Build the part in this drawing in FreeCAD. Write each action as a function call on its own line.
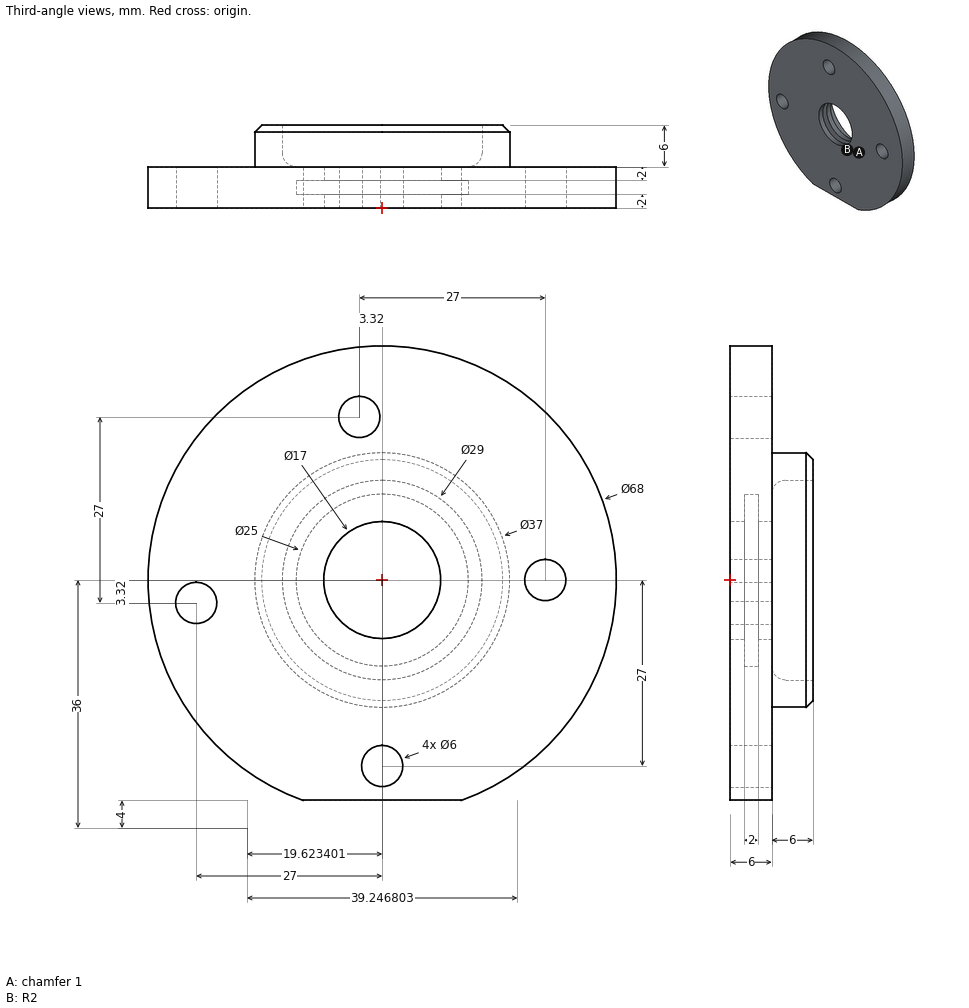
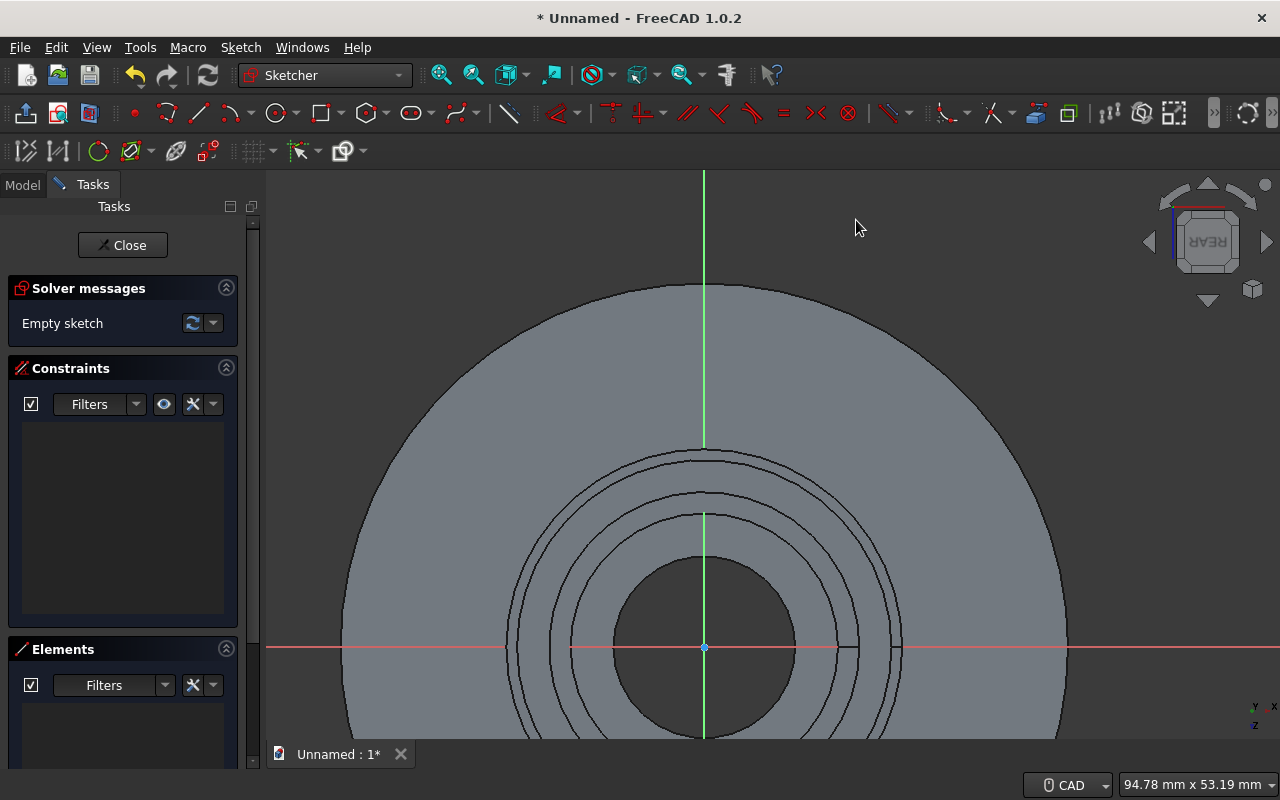
click(322, 114)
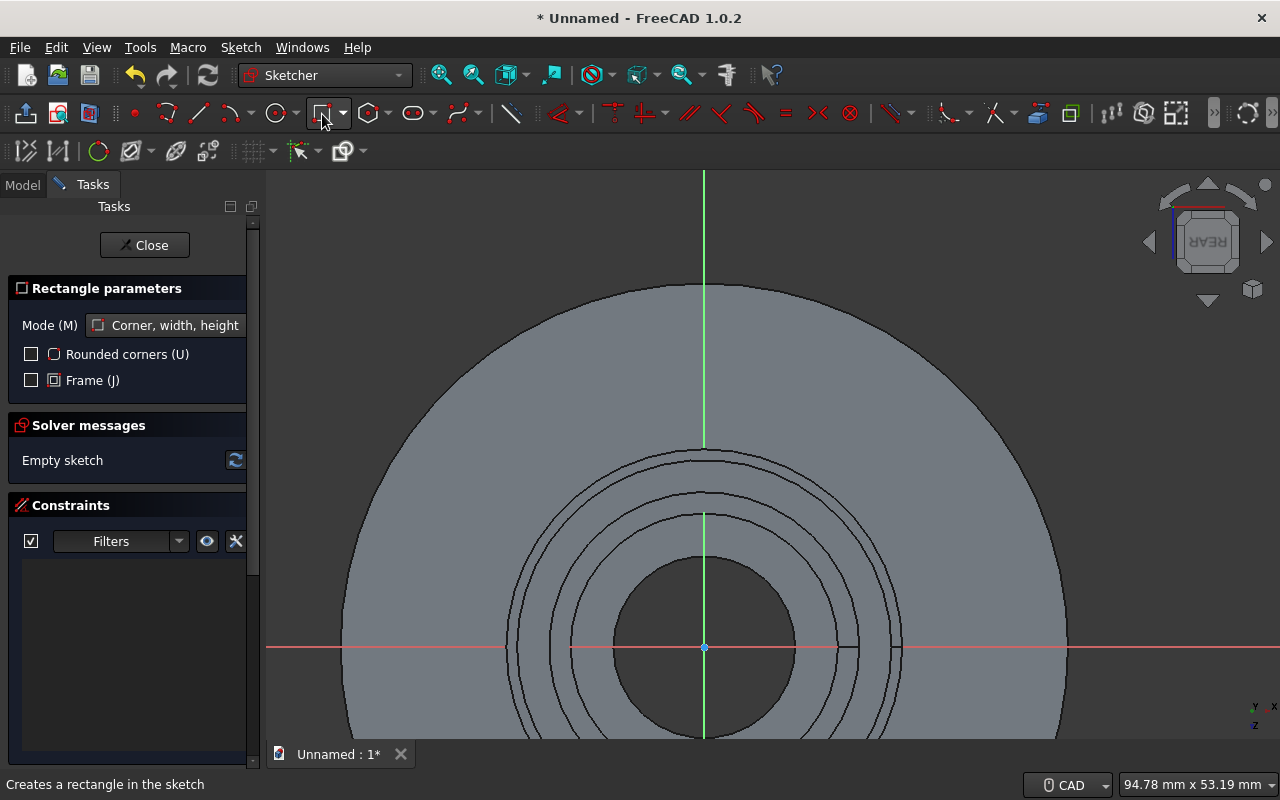
click(494, 262)
click(914, 305)
key(Escape)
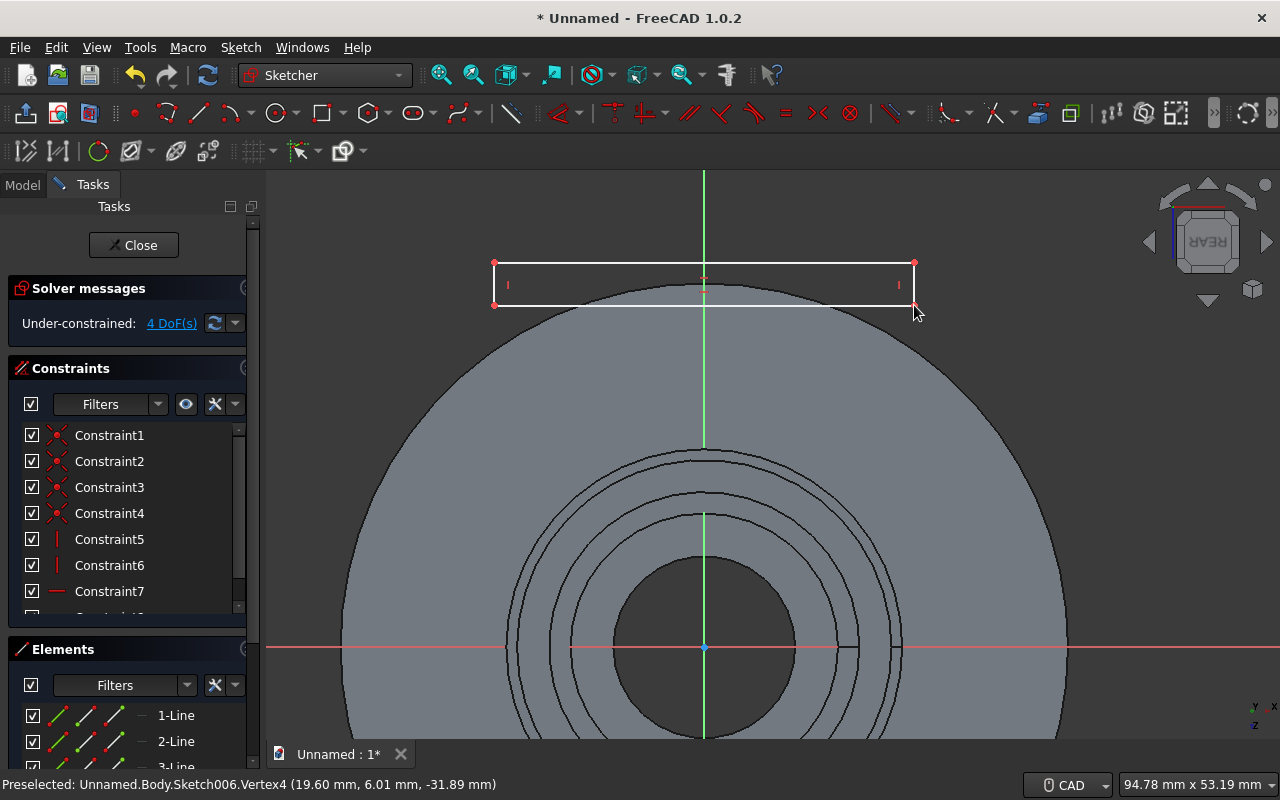
click(558, 114)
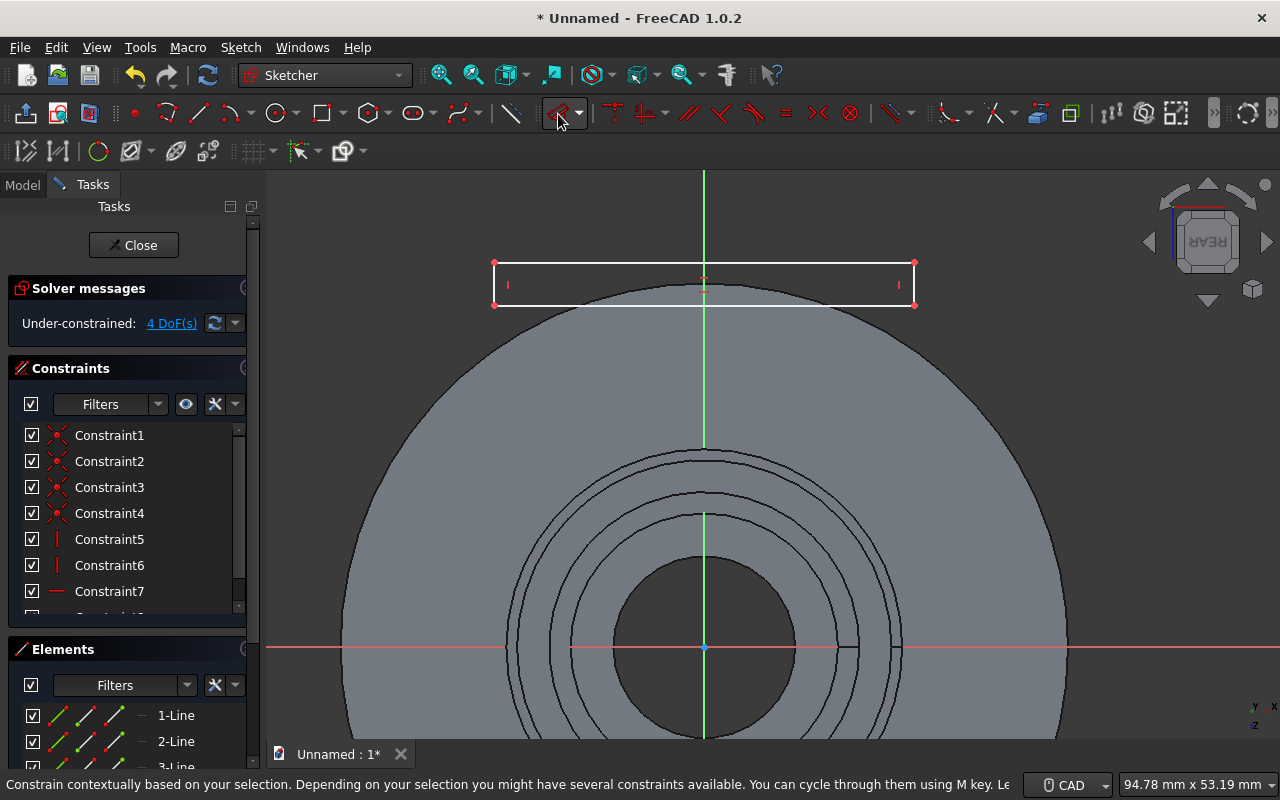
click(494, 276)
click(460, 285)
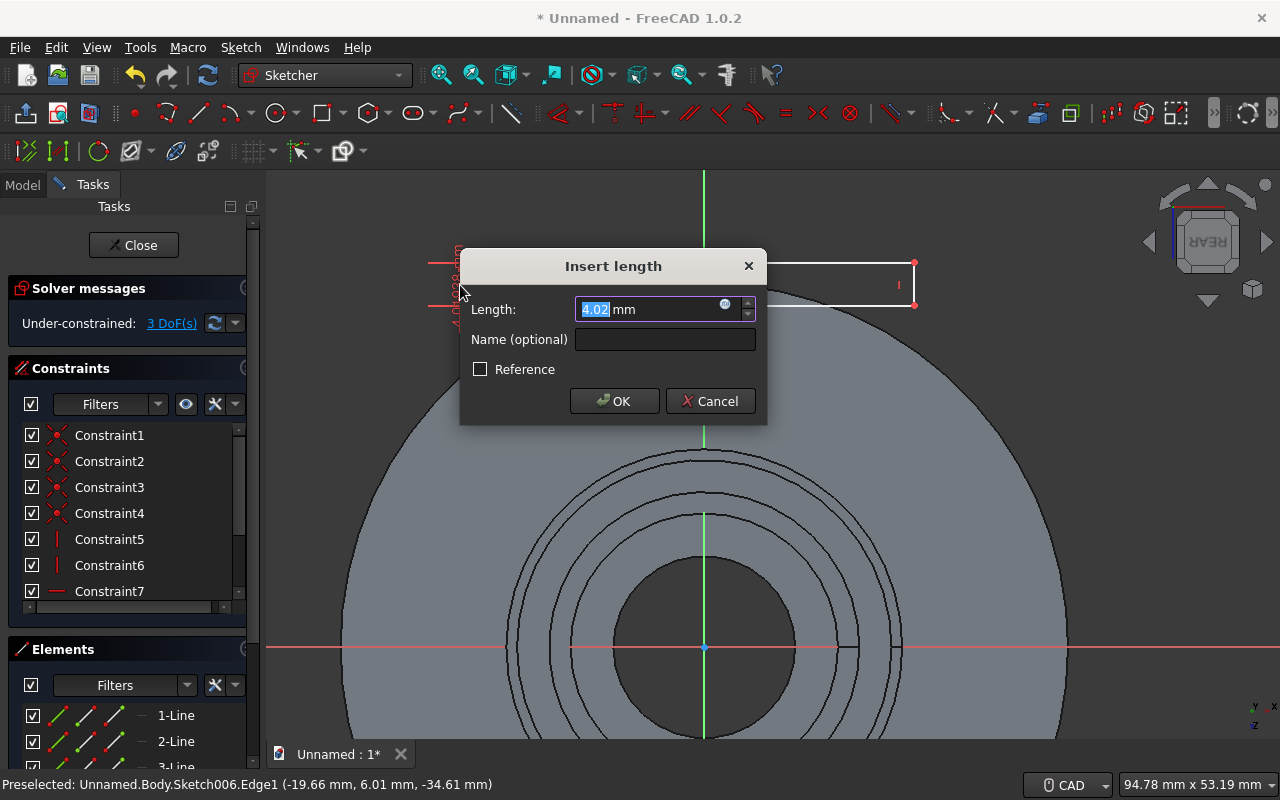
text(4)
key(Return)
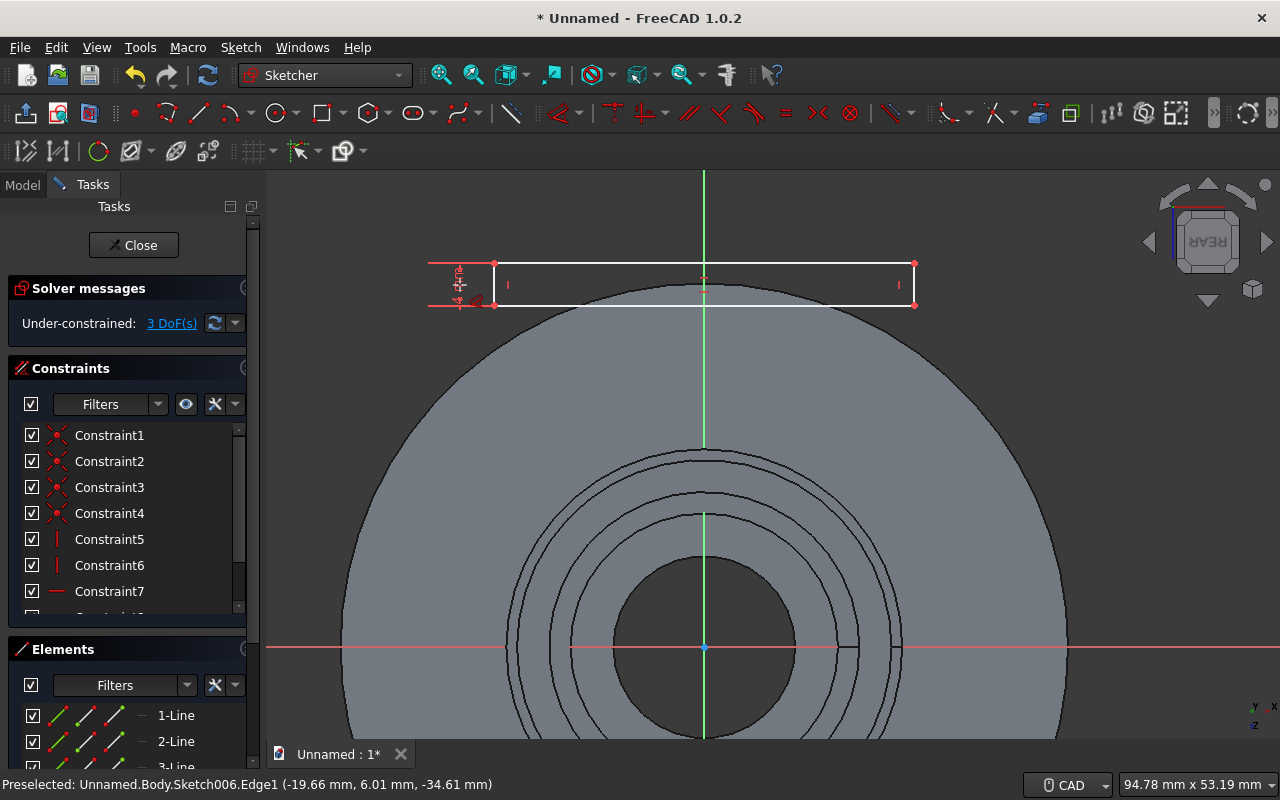
click(494, 263)
click(460, 455)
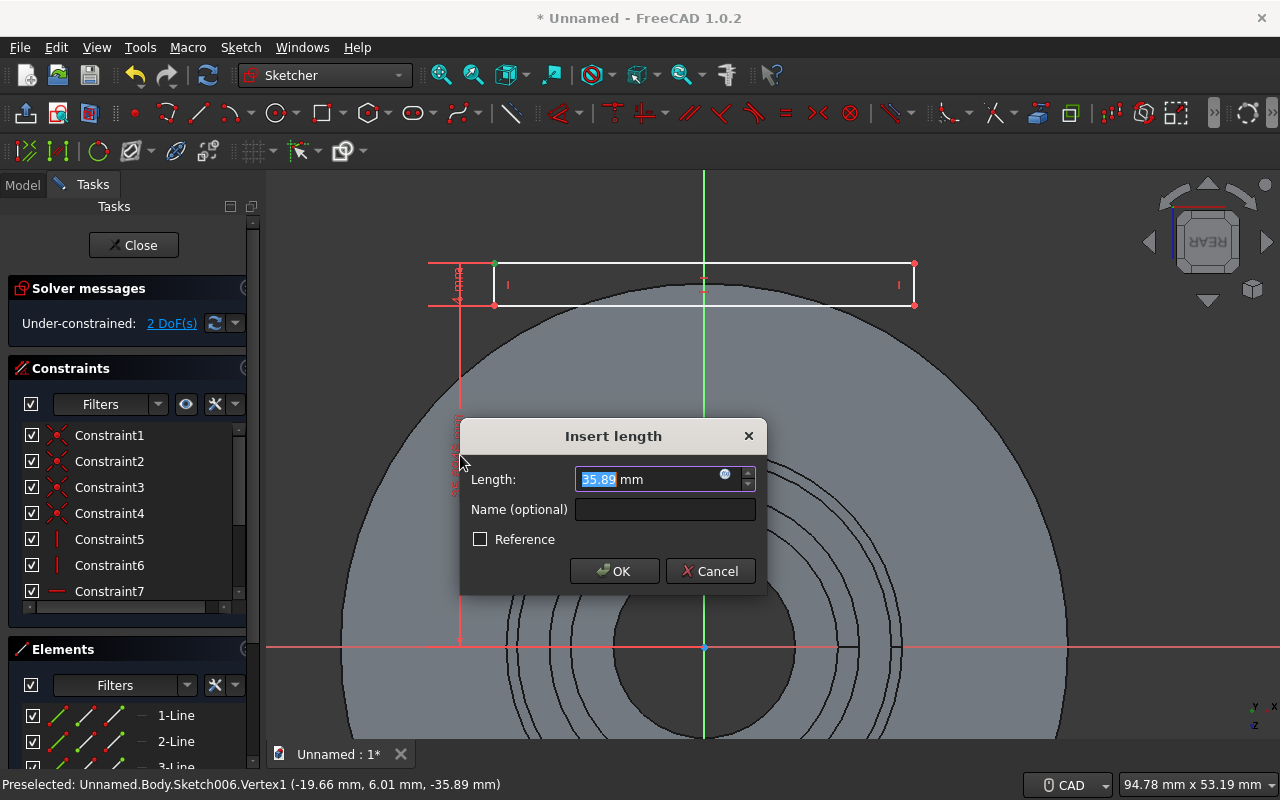
text(36)
key(Return)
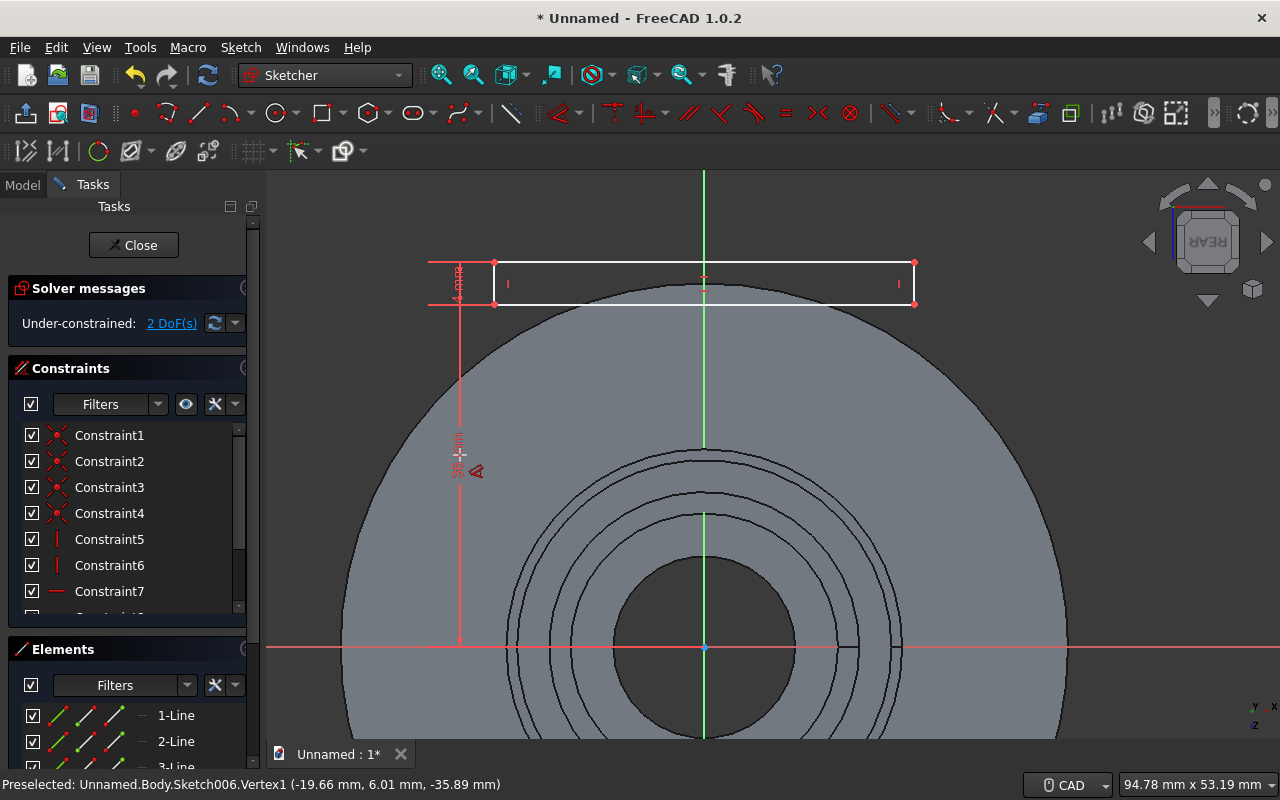
click(620, 305)
click(607, 339)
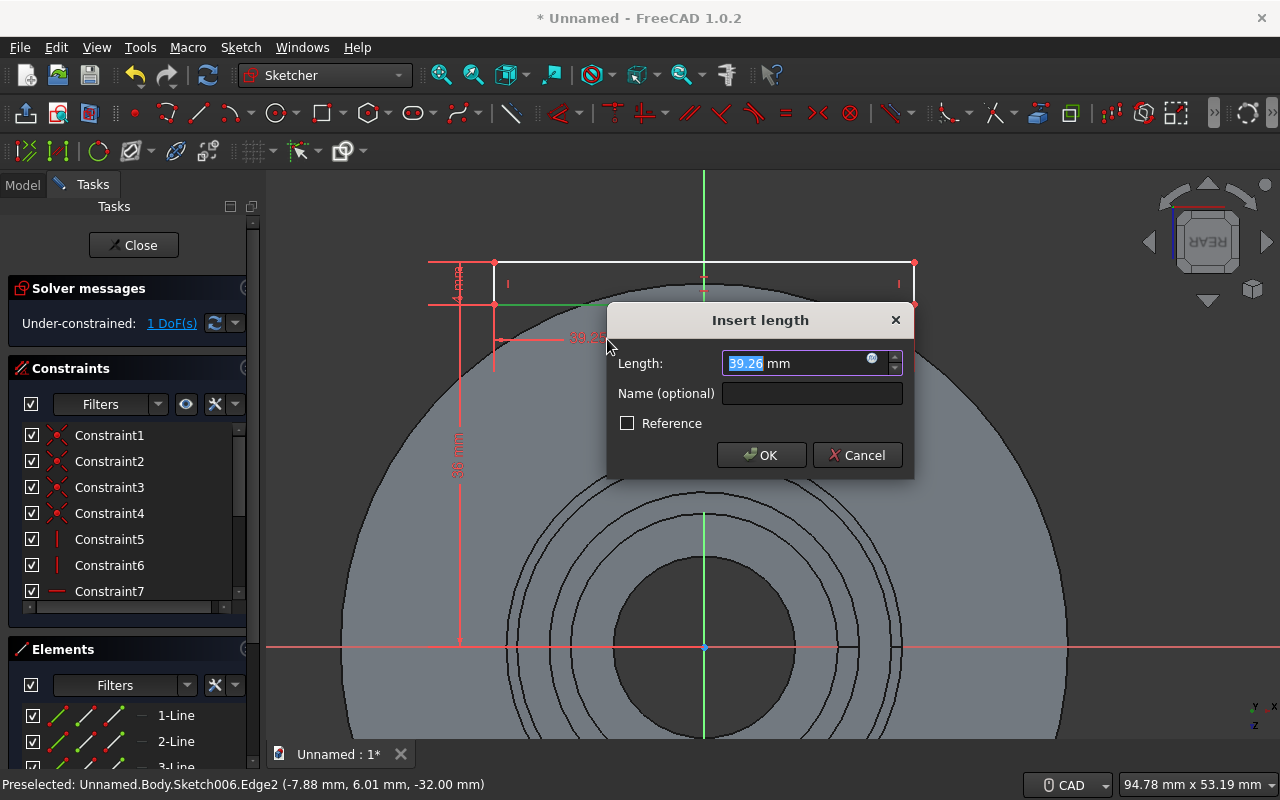
text(39.246803)
key(Return)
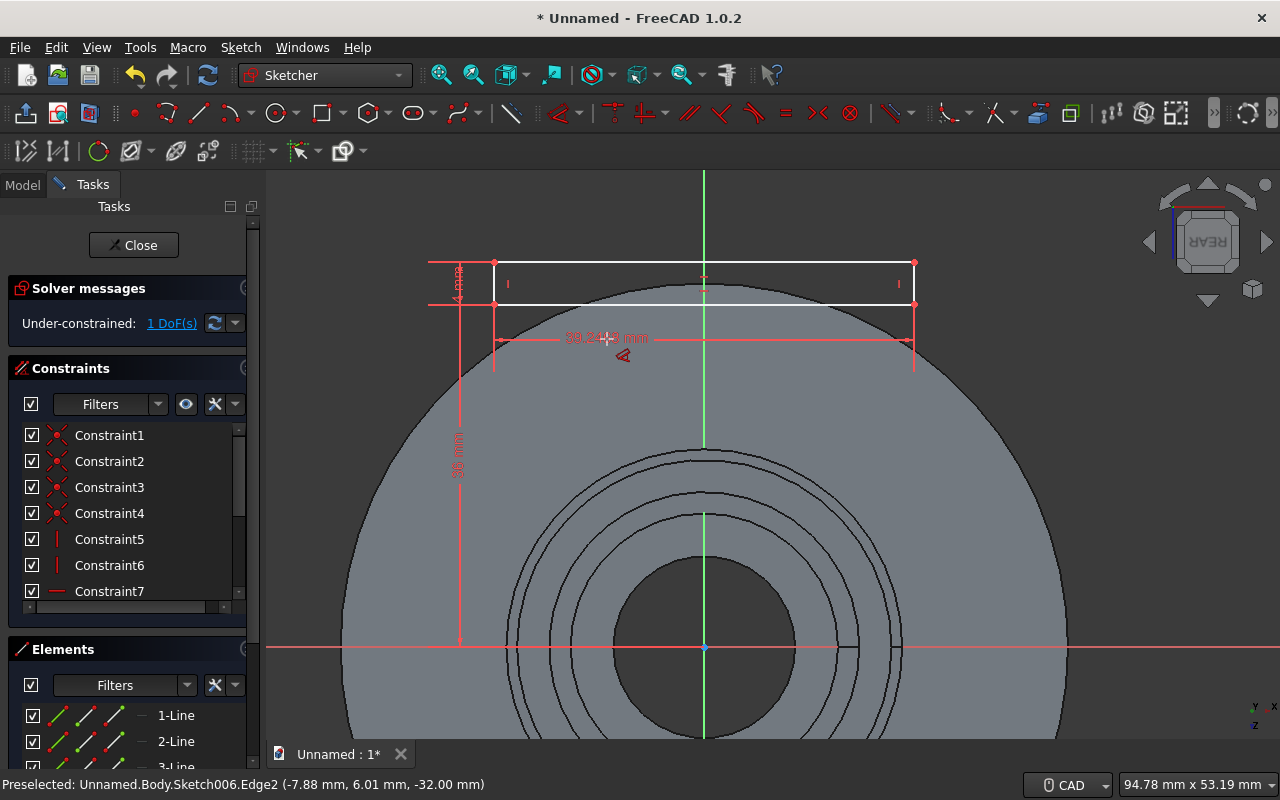
click(494, 262)
click(599, 681)